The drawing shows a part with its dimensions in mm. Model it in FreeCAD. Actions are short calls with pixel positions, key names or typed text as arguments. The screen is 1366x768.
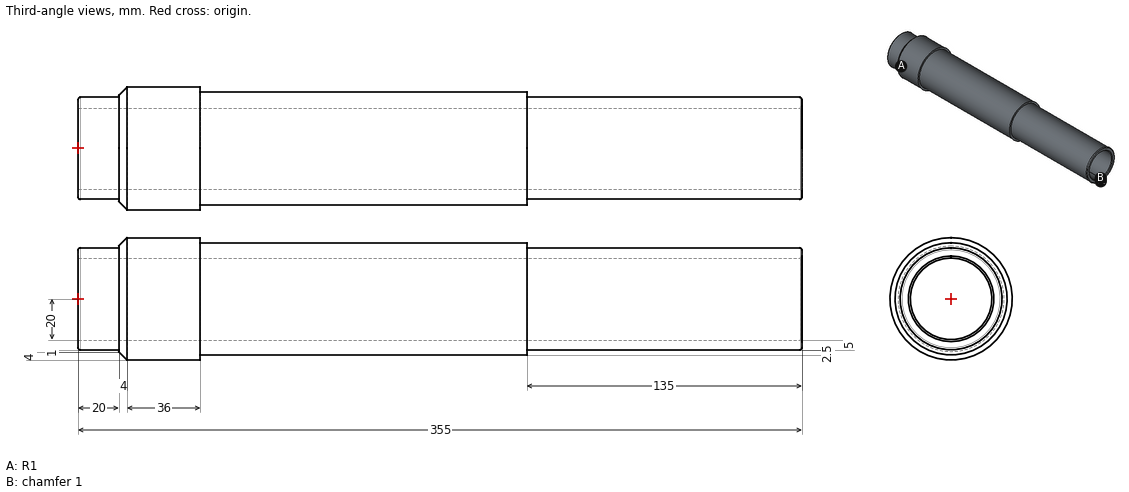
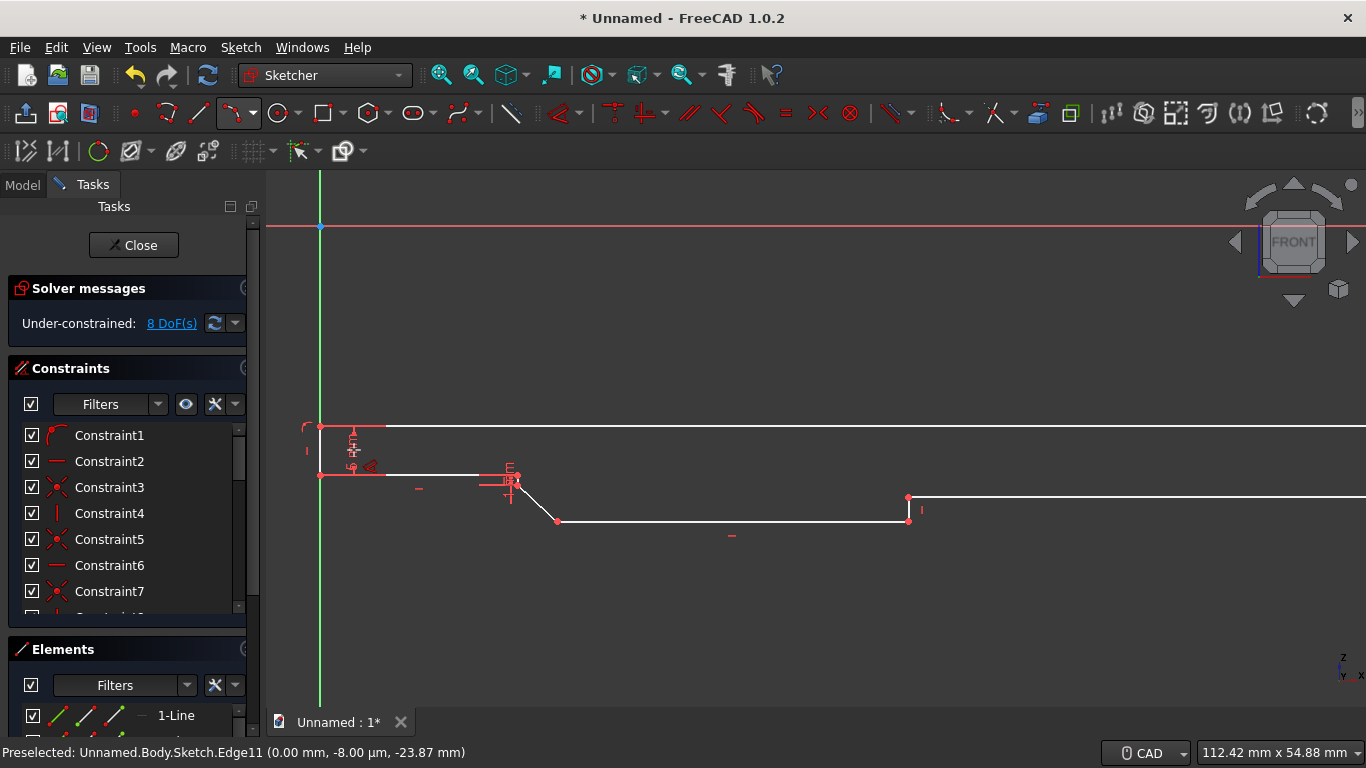
scroll(416, 455, down, 8)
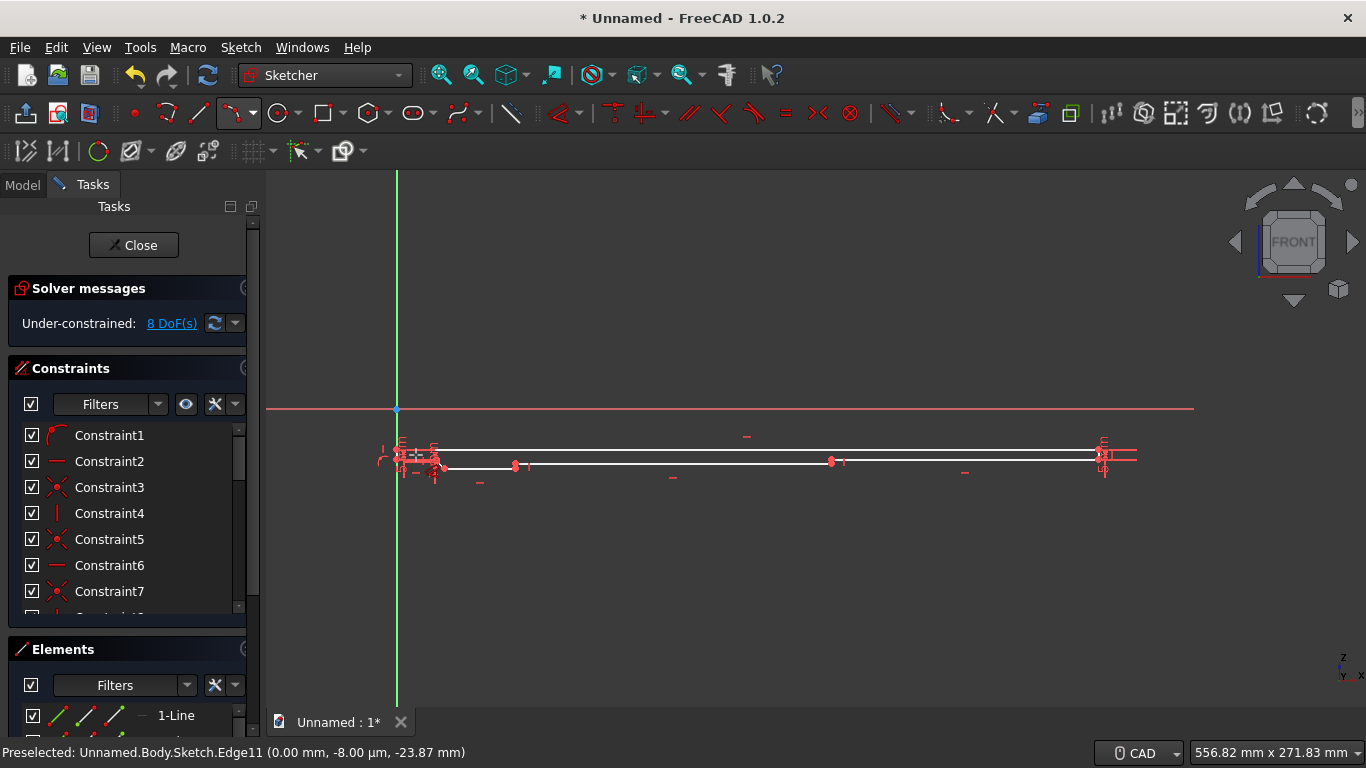
click(494, 469)
click(480, 503)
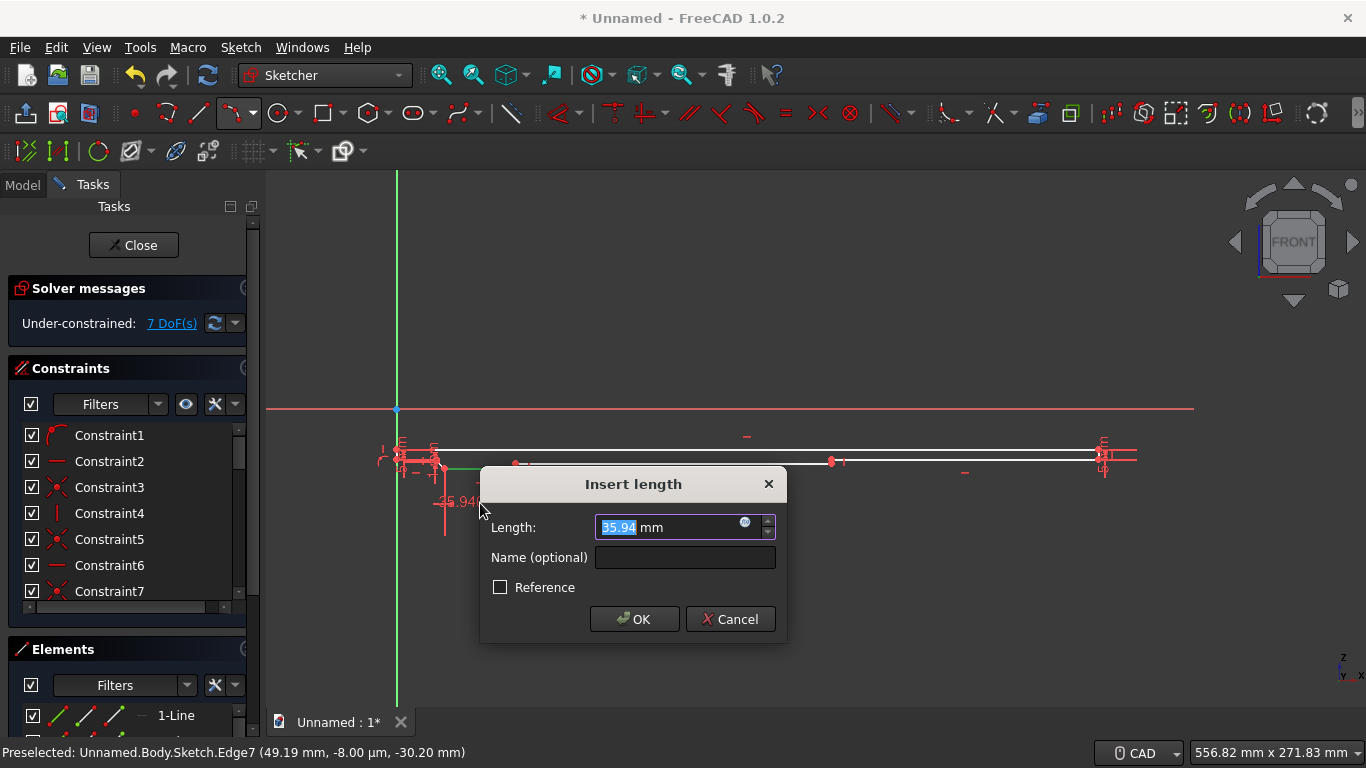
text(36)
key(Return)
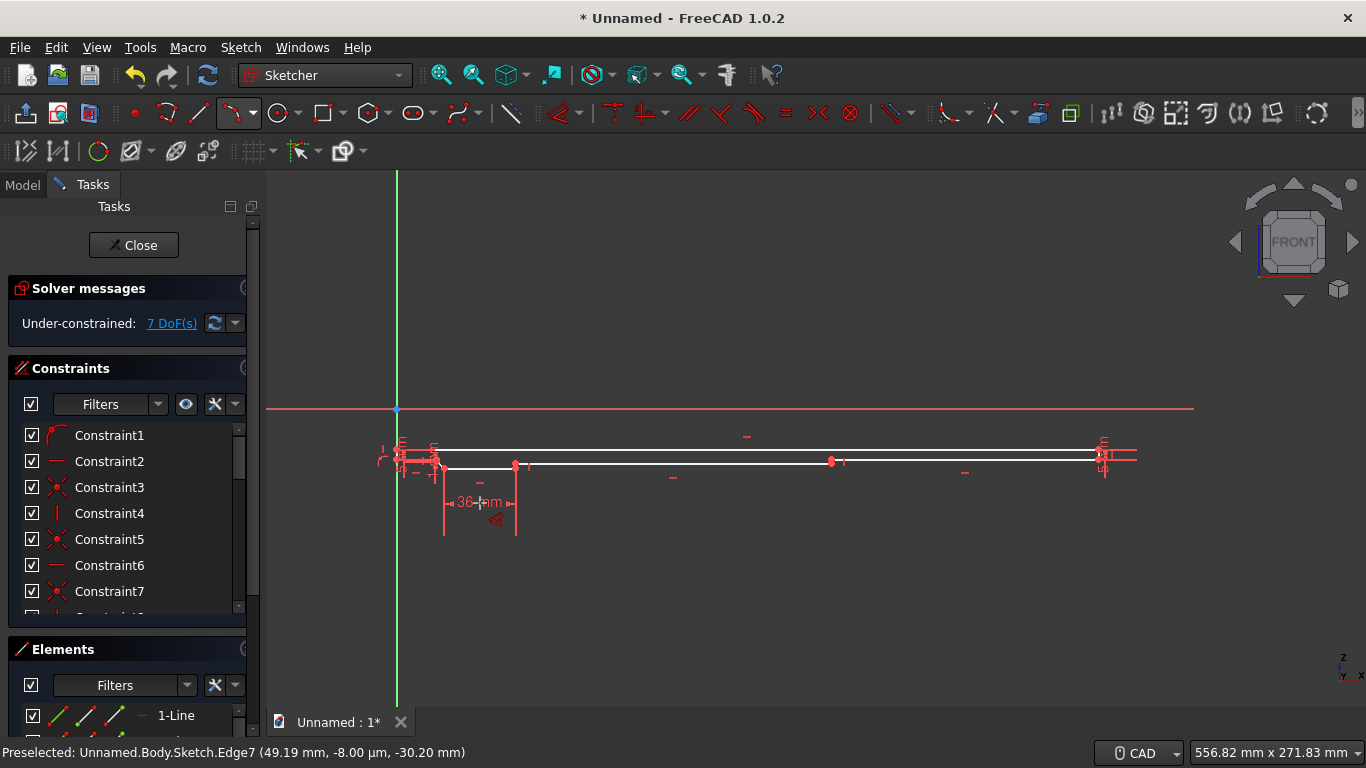
scroll(425, 460, up, 2)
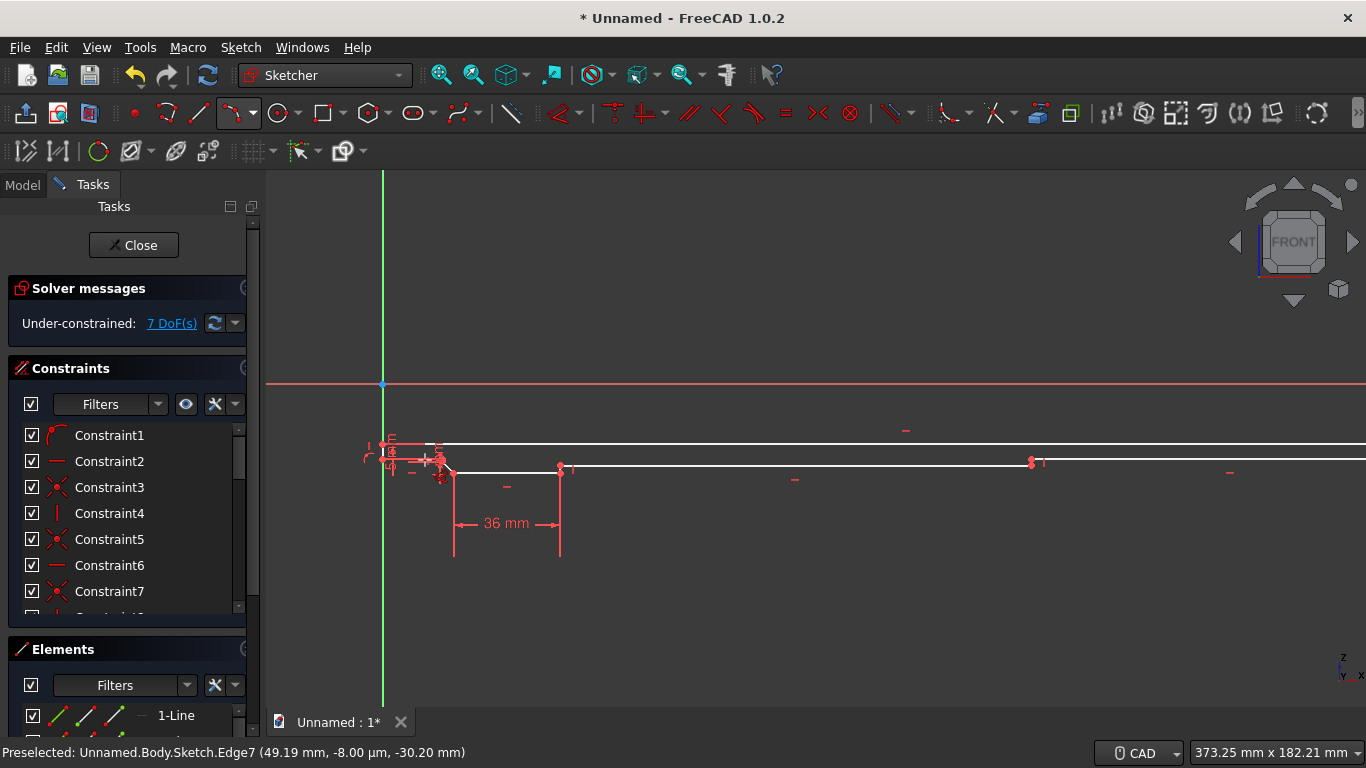
click(424, 459)
click(413, 493)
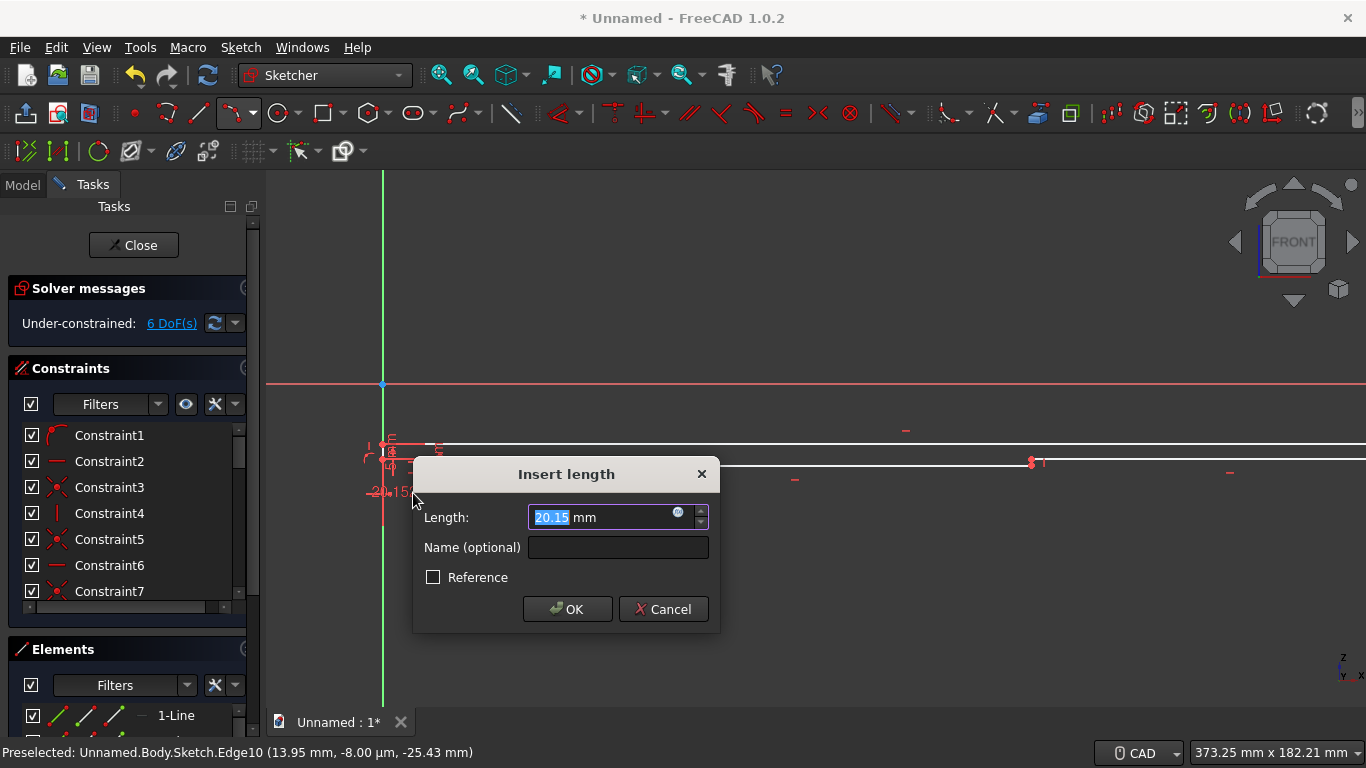
text(20)
key(Return)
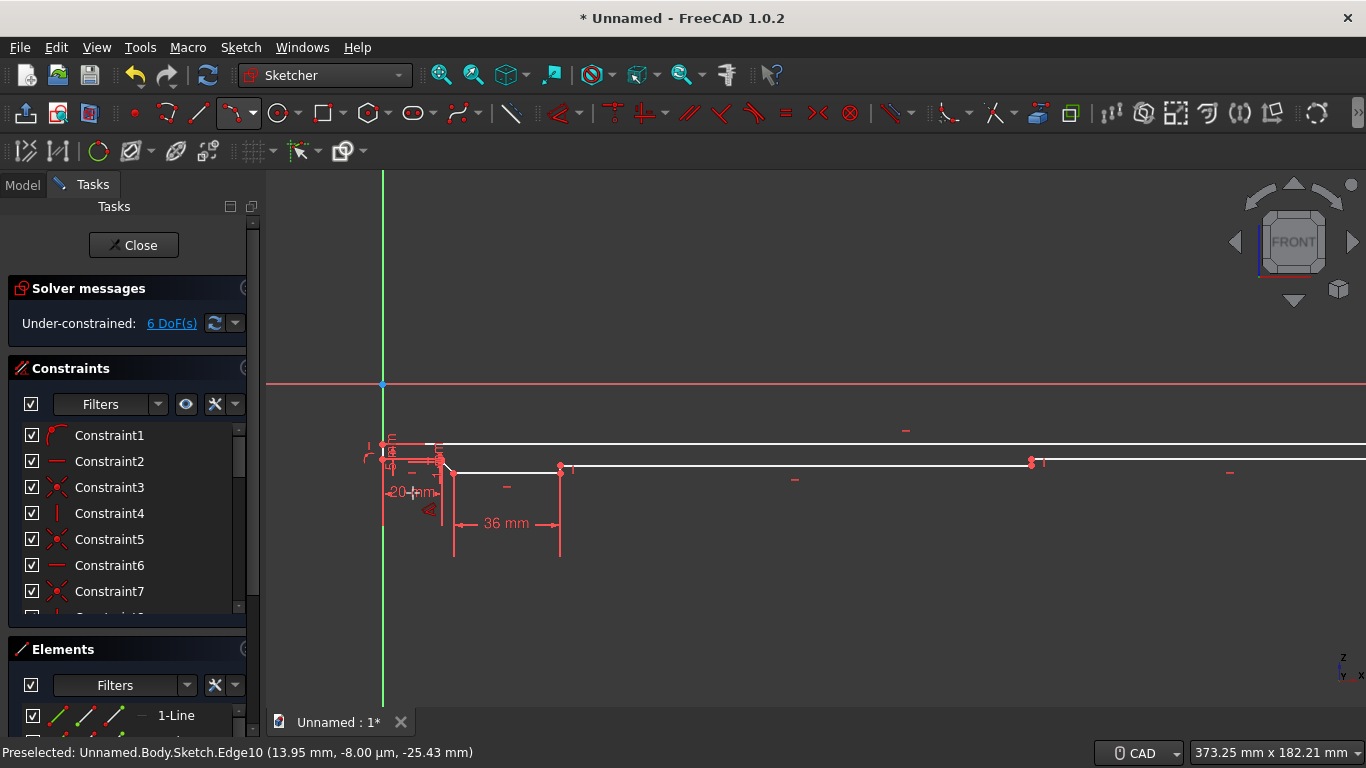
scroll(448, 468, up, 7)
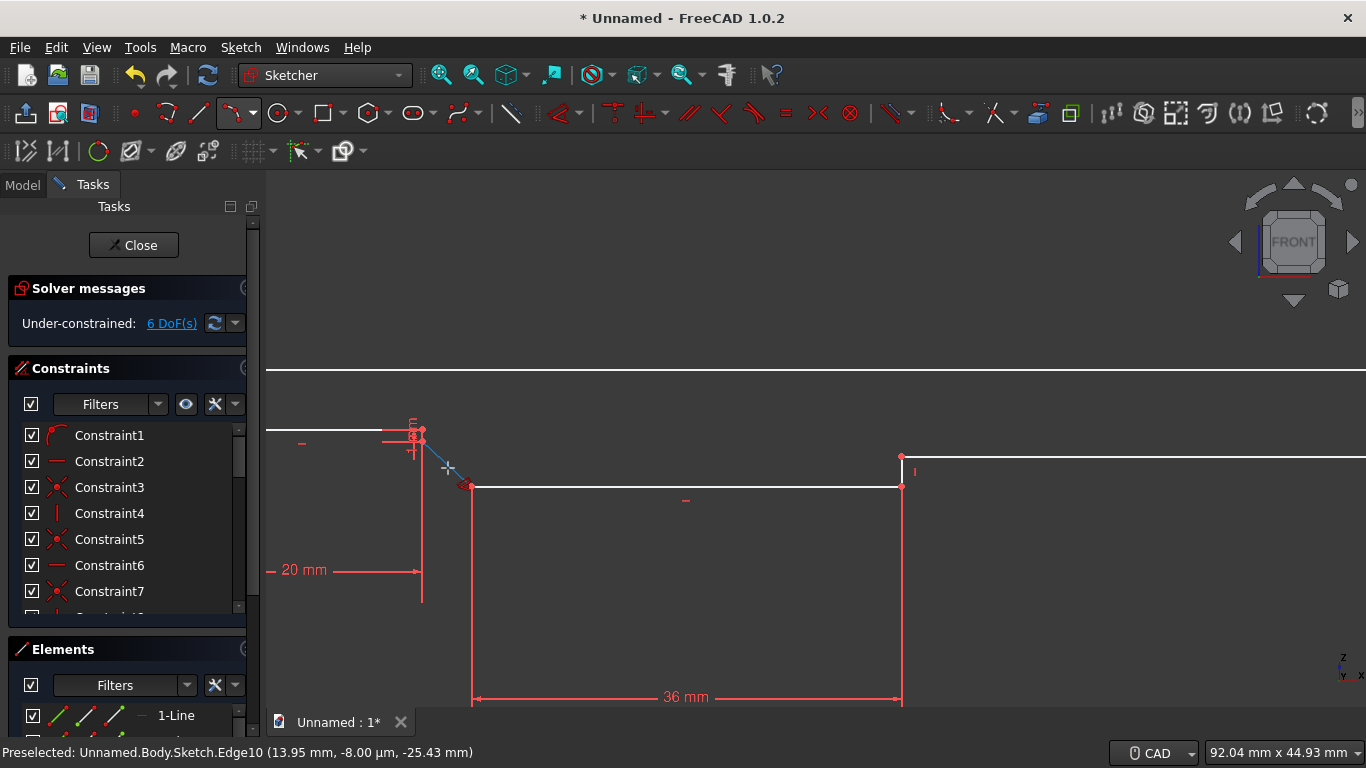
click(447, 464)
click(447, 521)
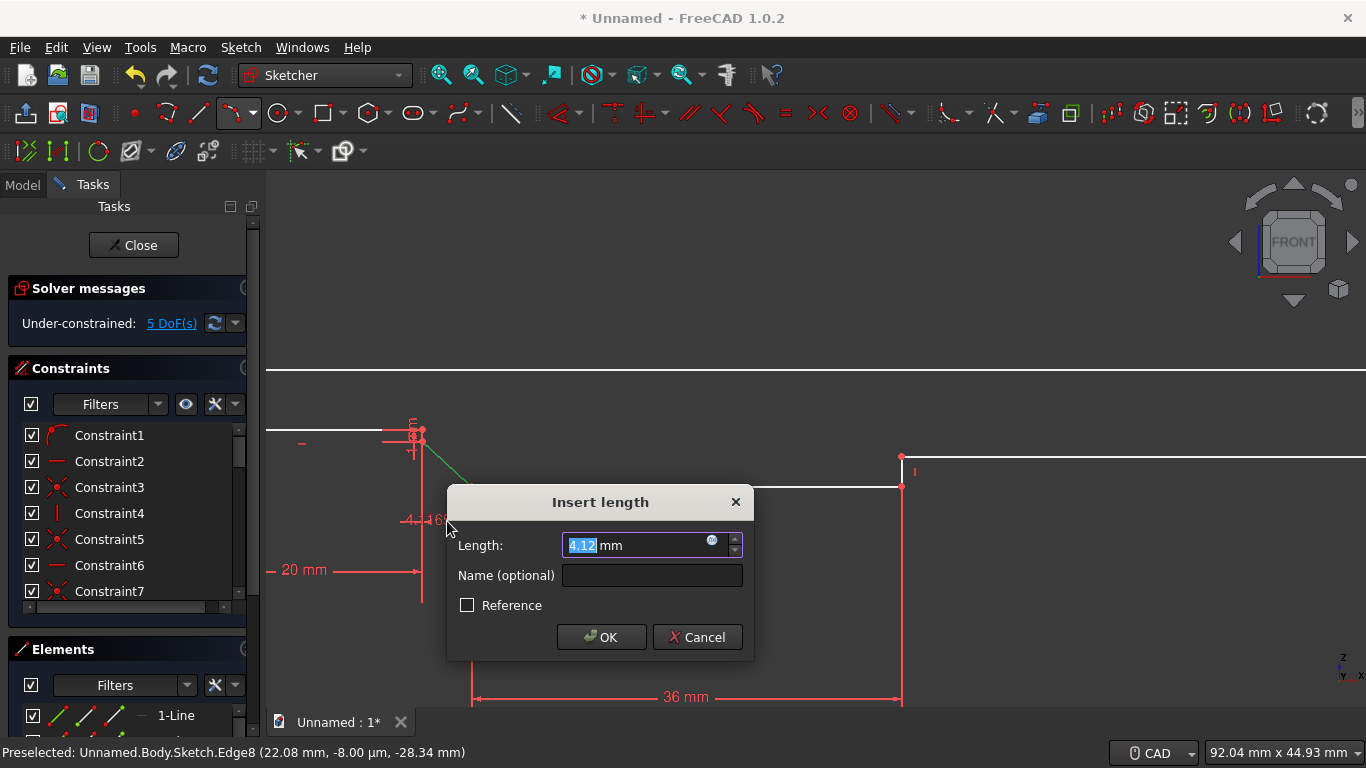
text(4)
key(Return)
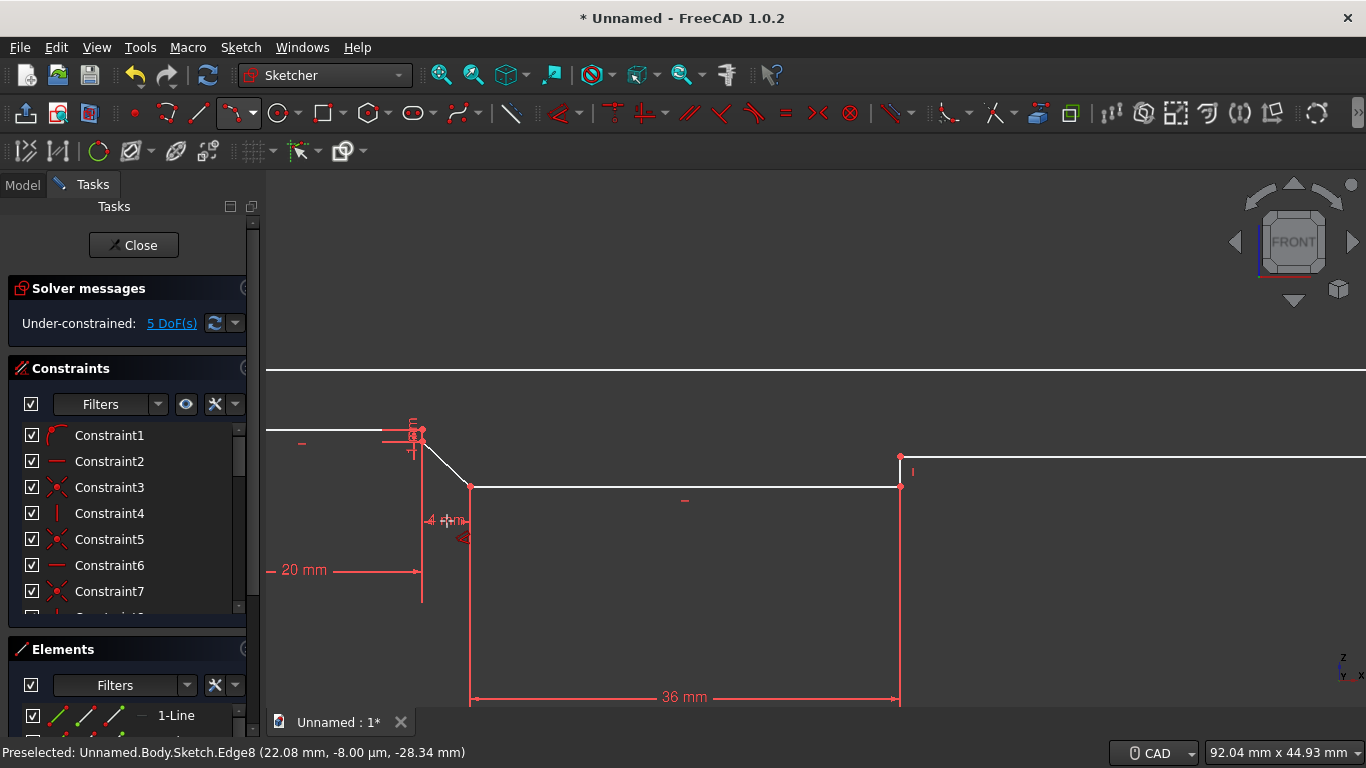
click(456, 473)
click(388, 464)